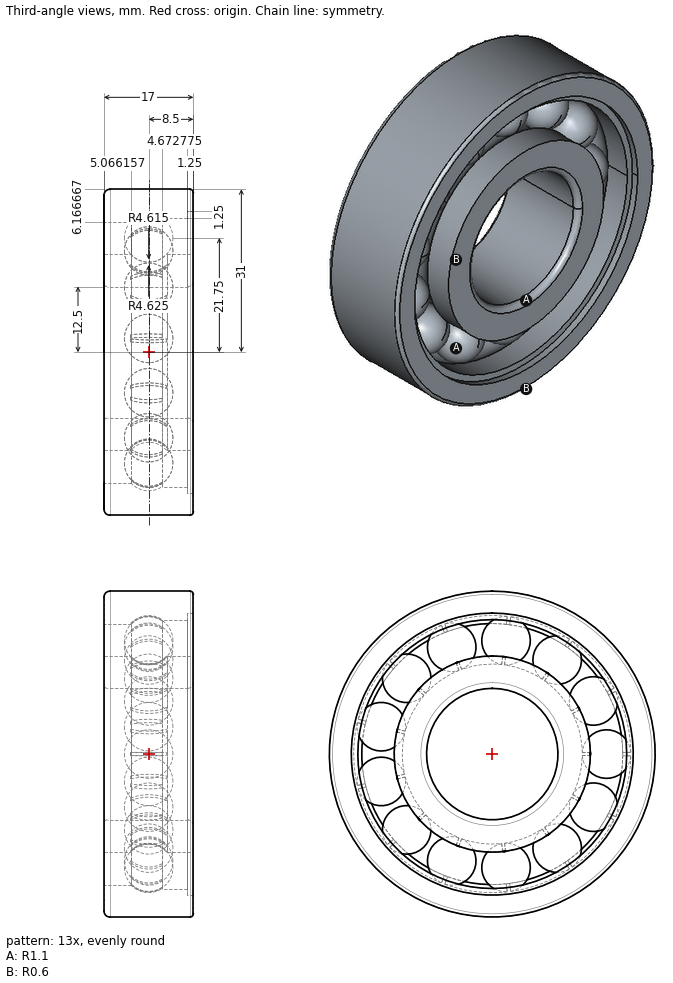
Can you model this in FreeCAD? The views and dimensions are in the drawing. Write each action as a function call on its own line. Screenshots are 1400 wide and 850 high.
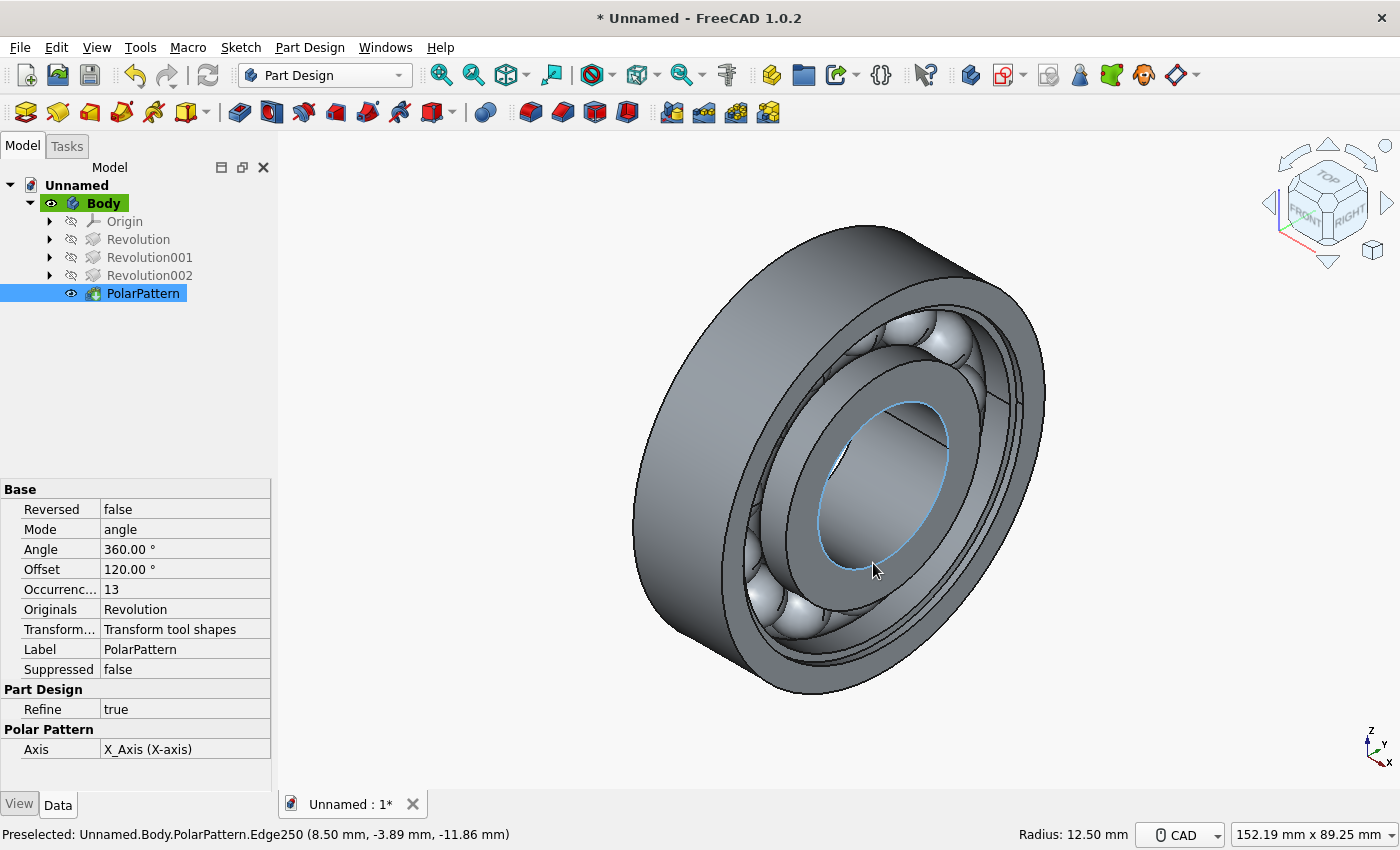
key(2)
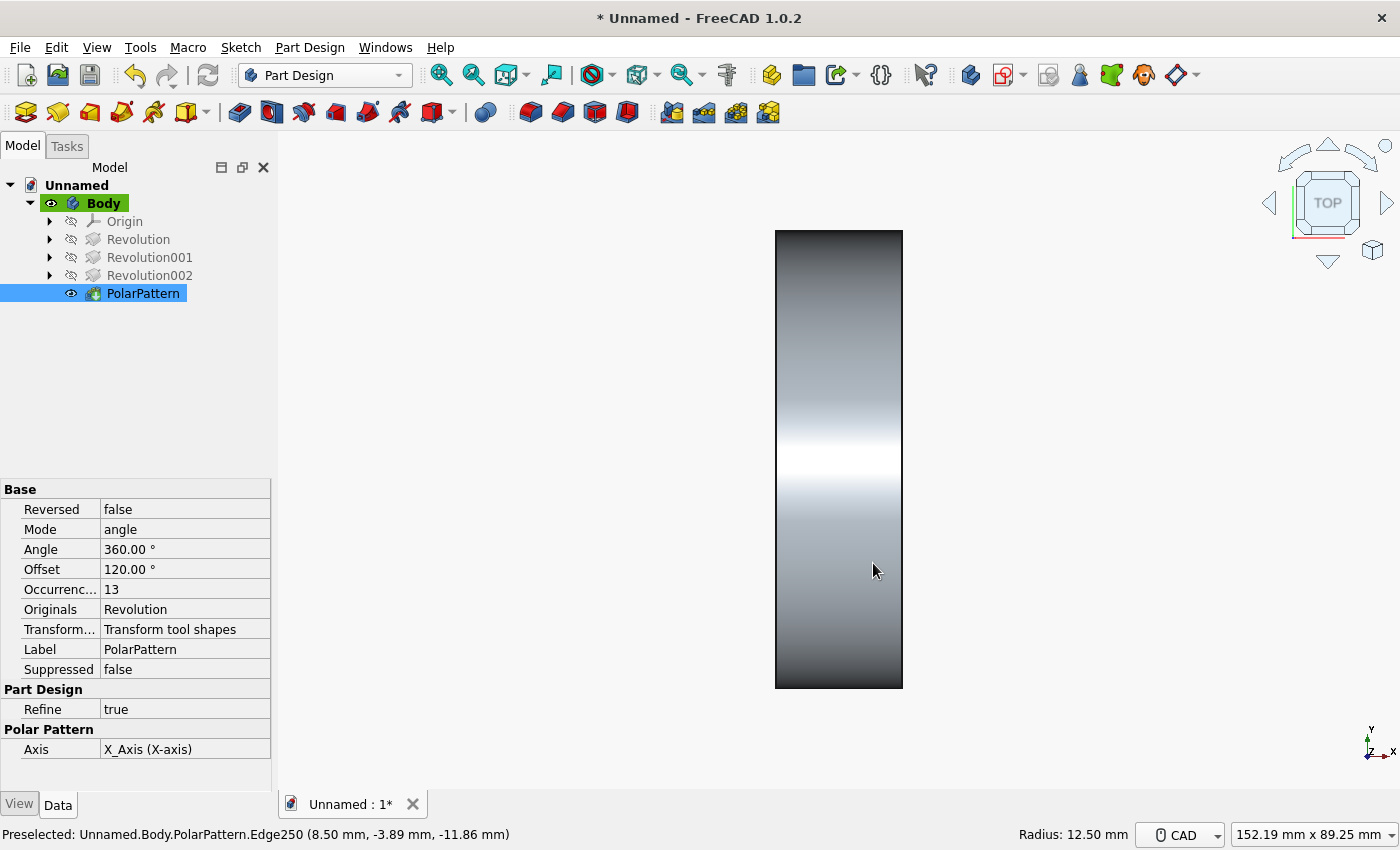
click(776, 644, ctrl)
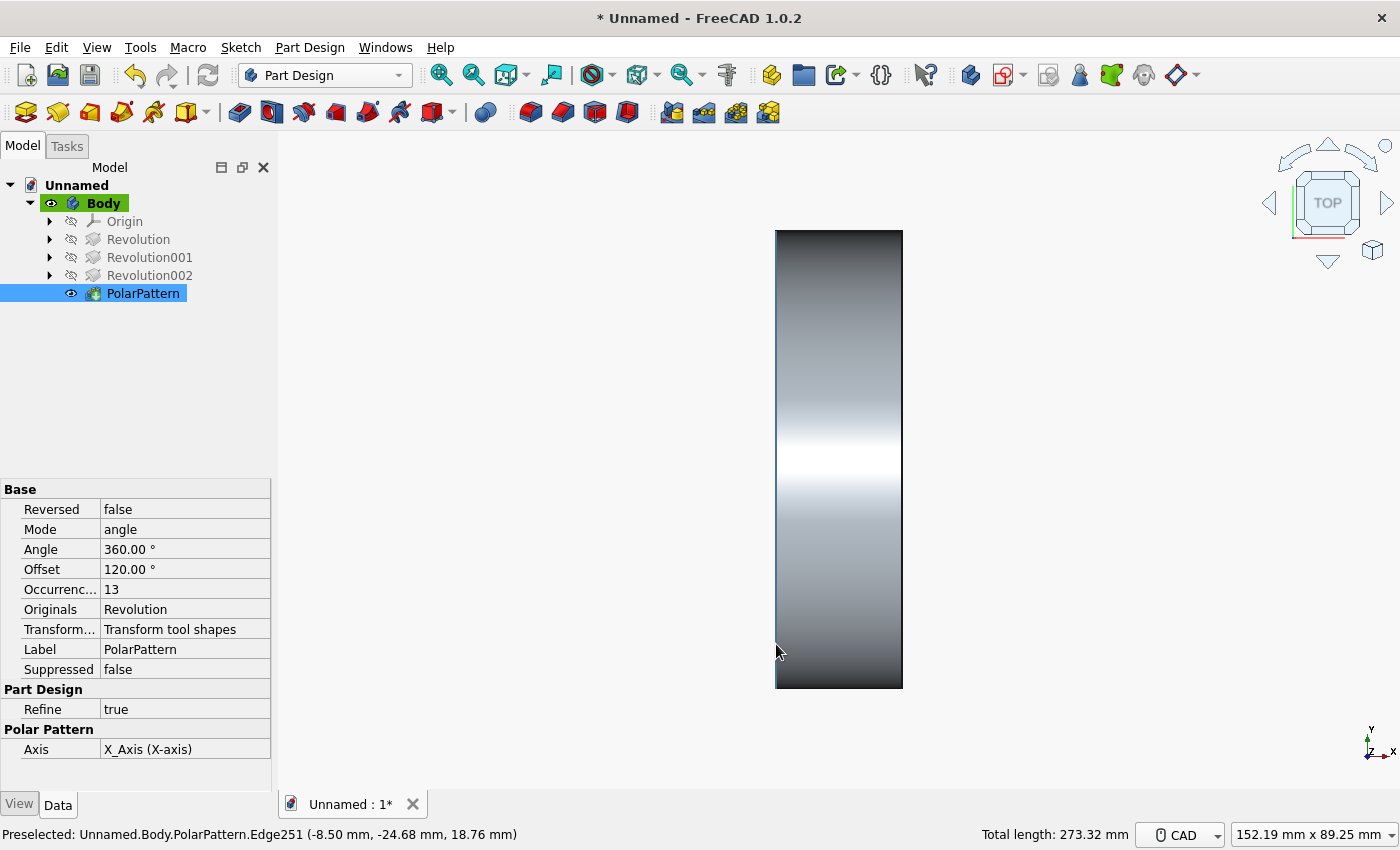
click(532, 112)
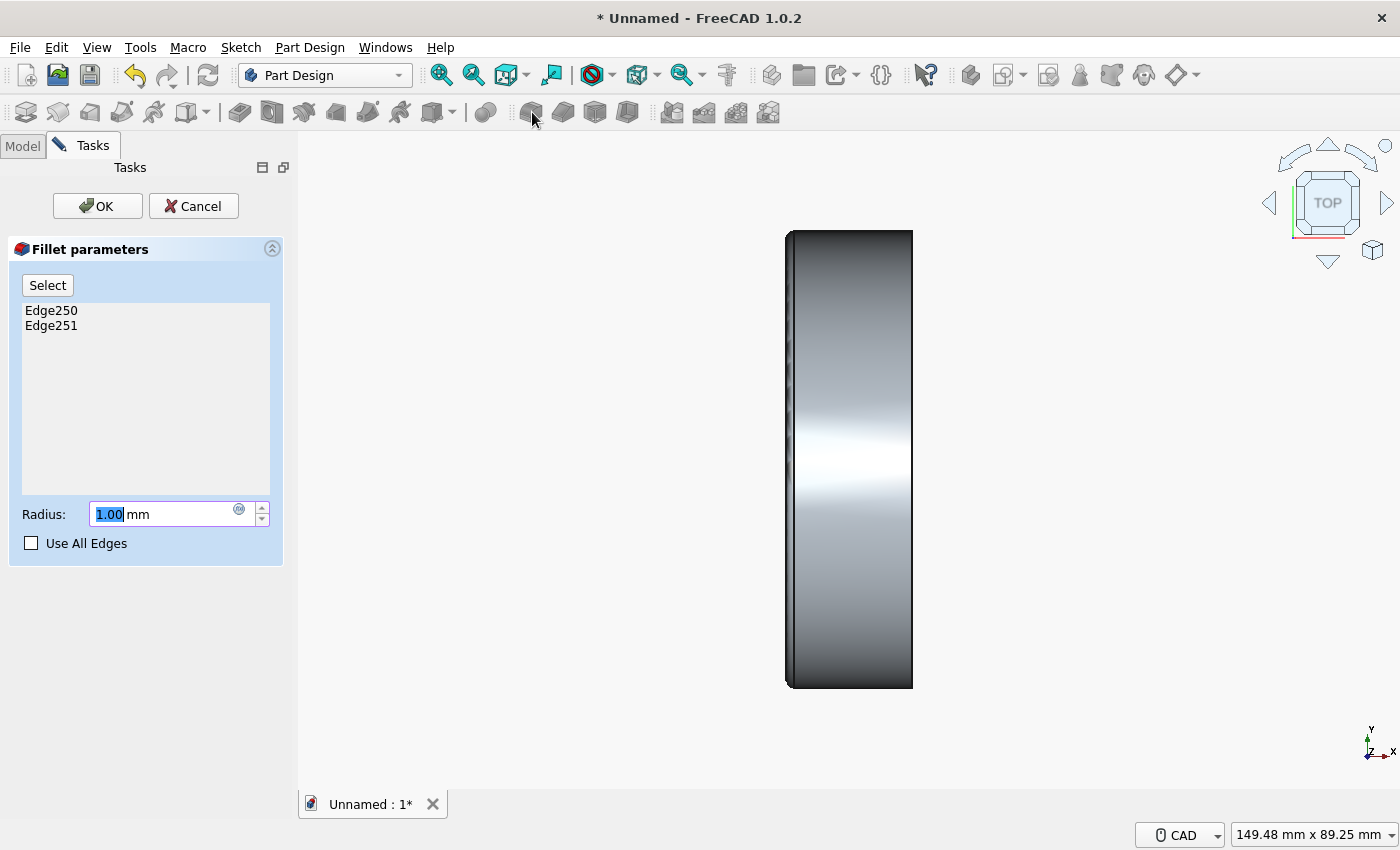
text(1.1)
key(Tab)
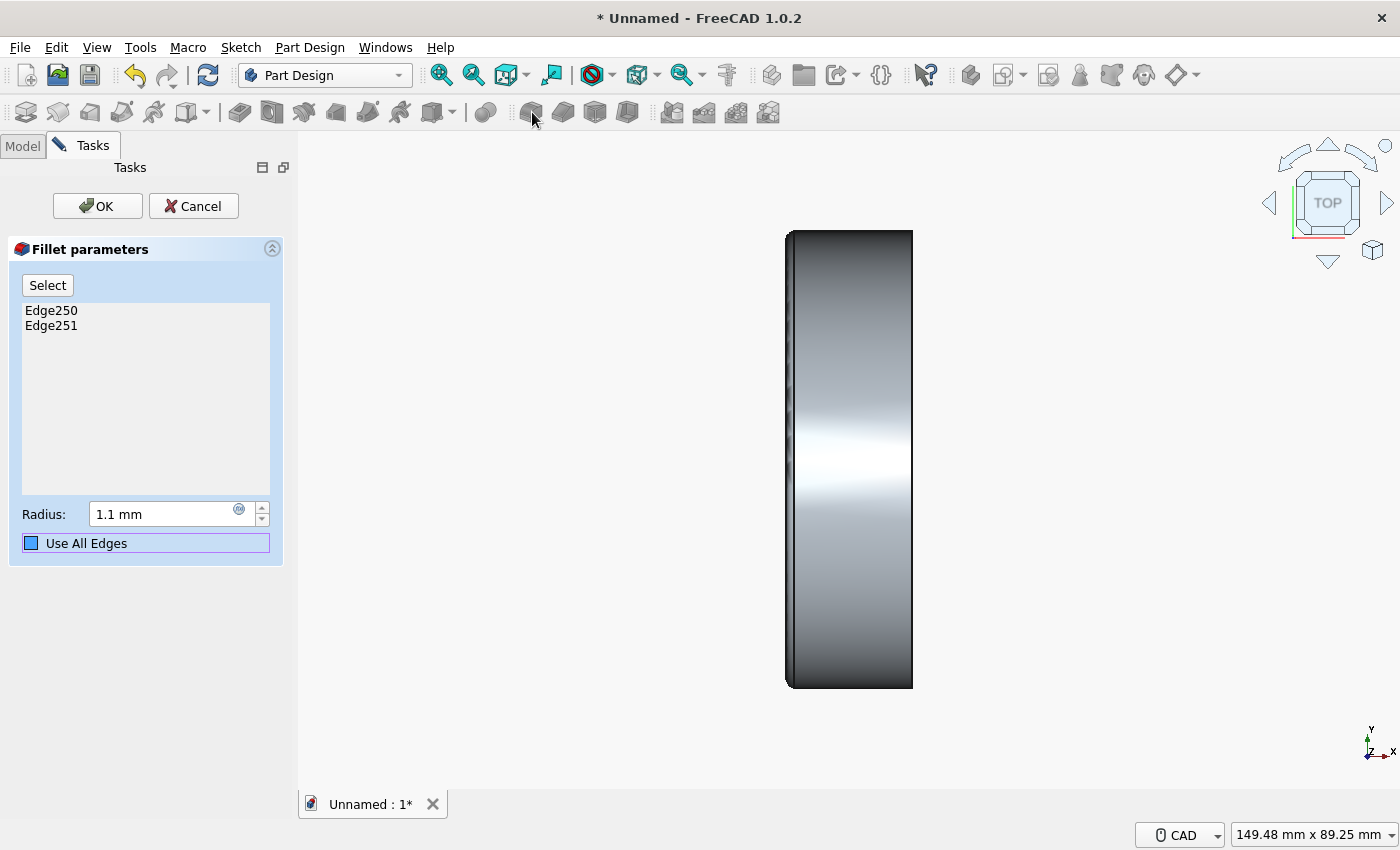
click(98, 206)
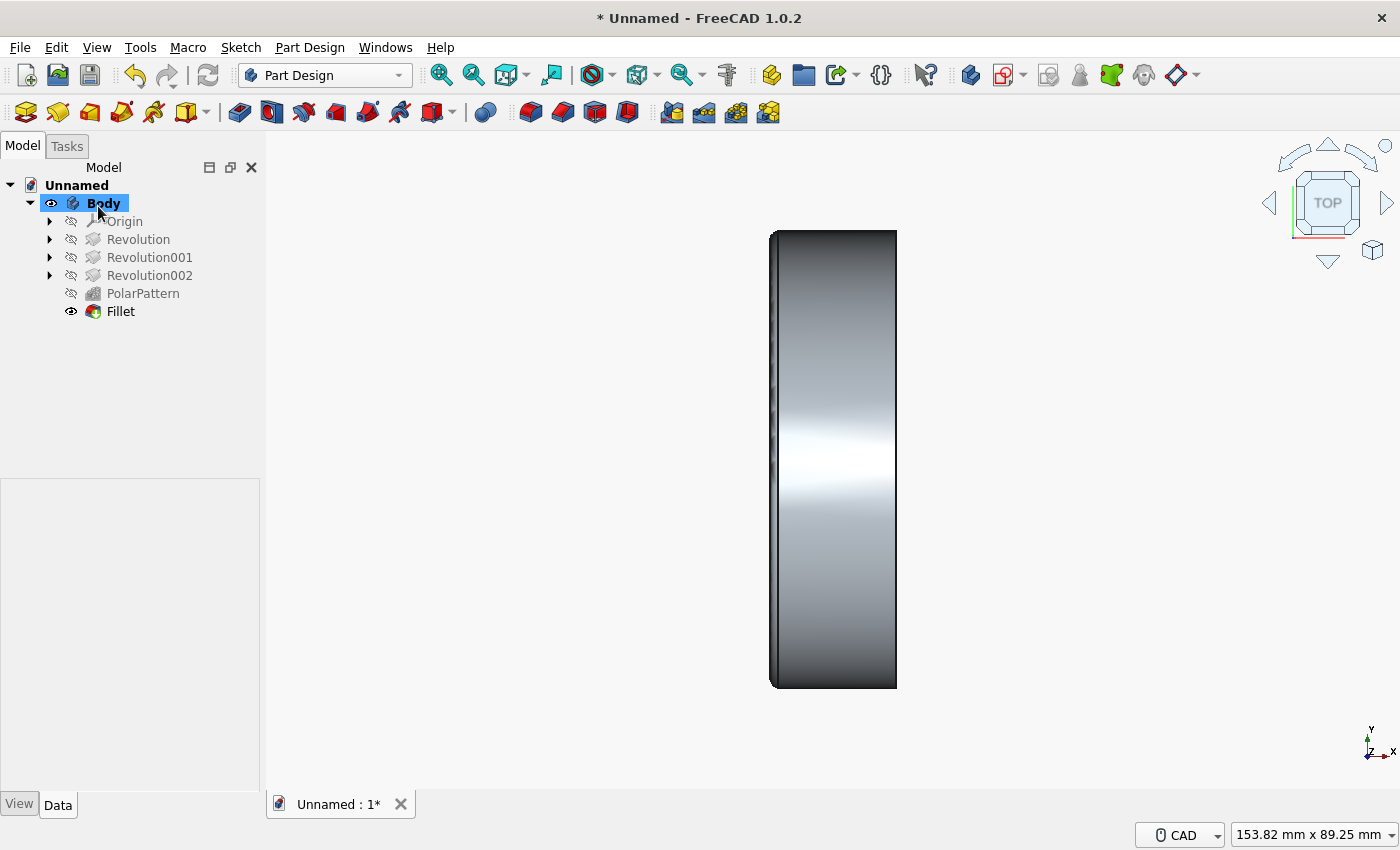
click(896, 292)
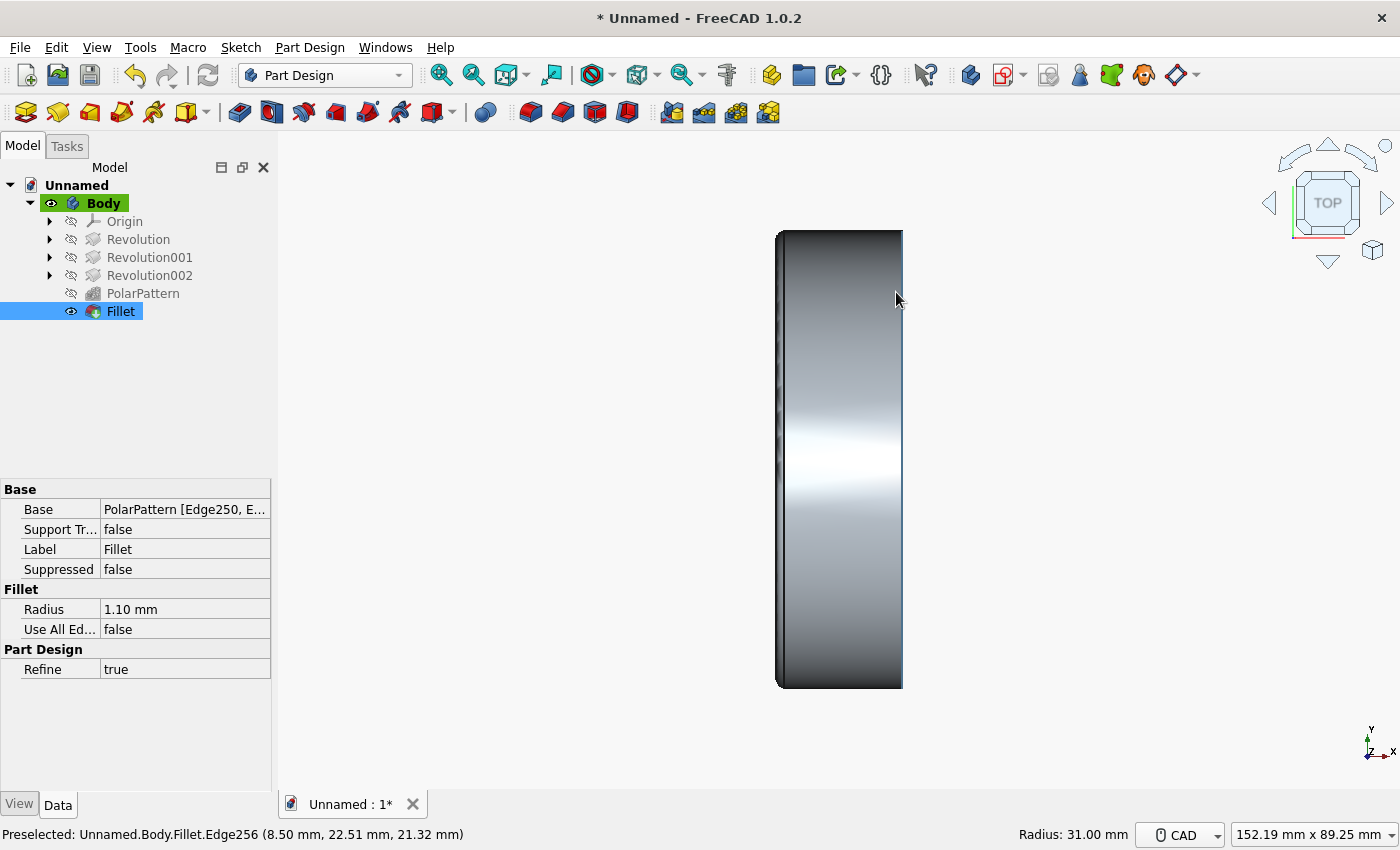
key(0)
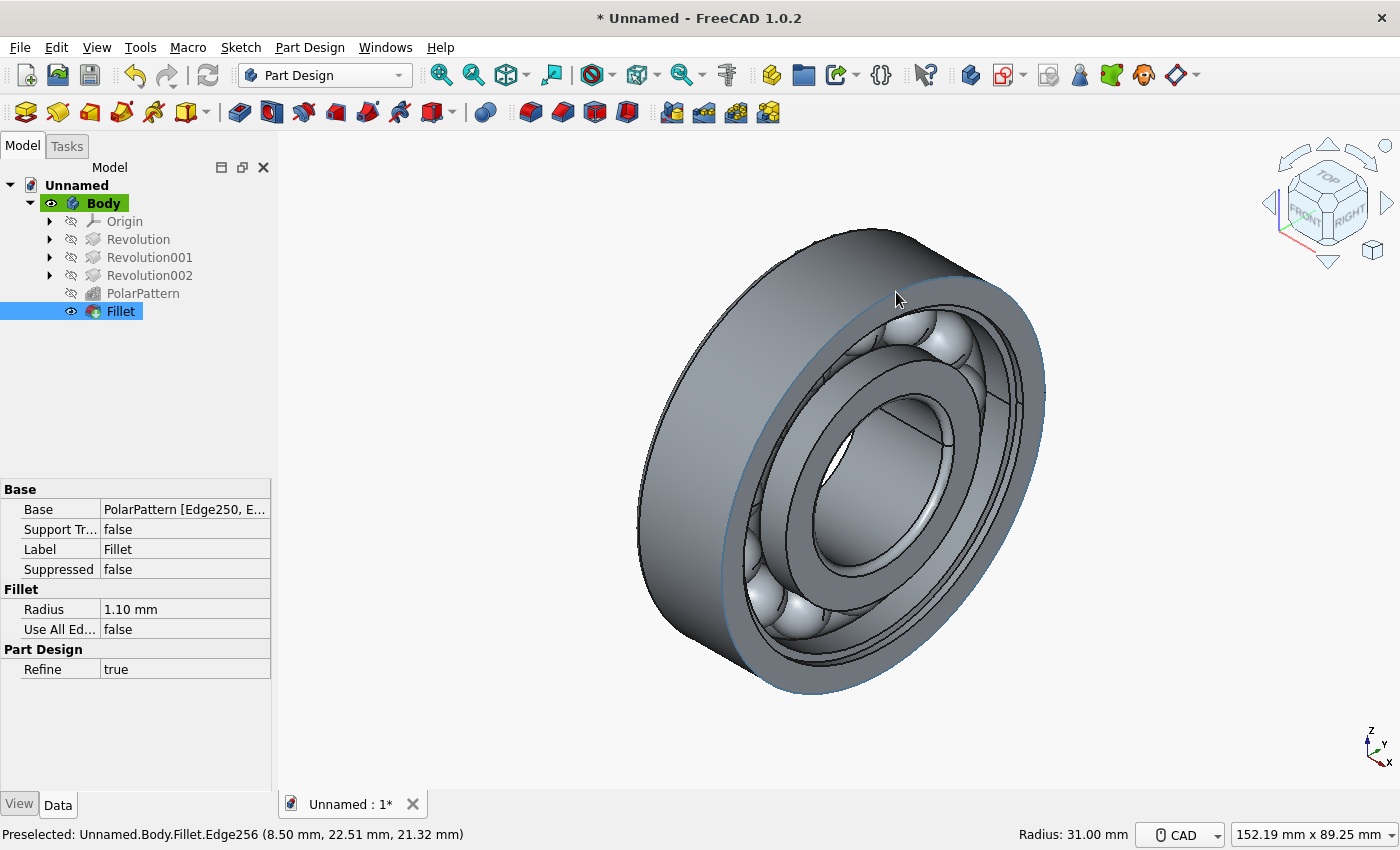
key(2)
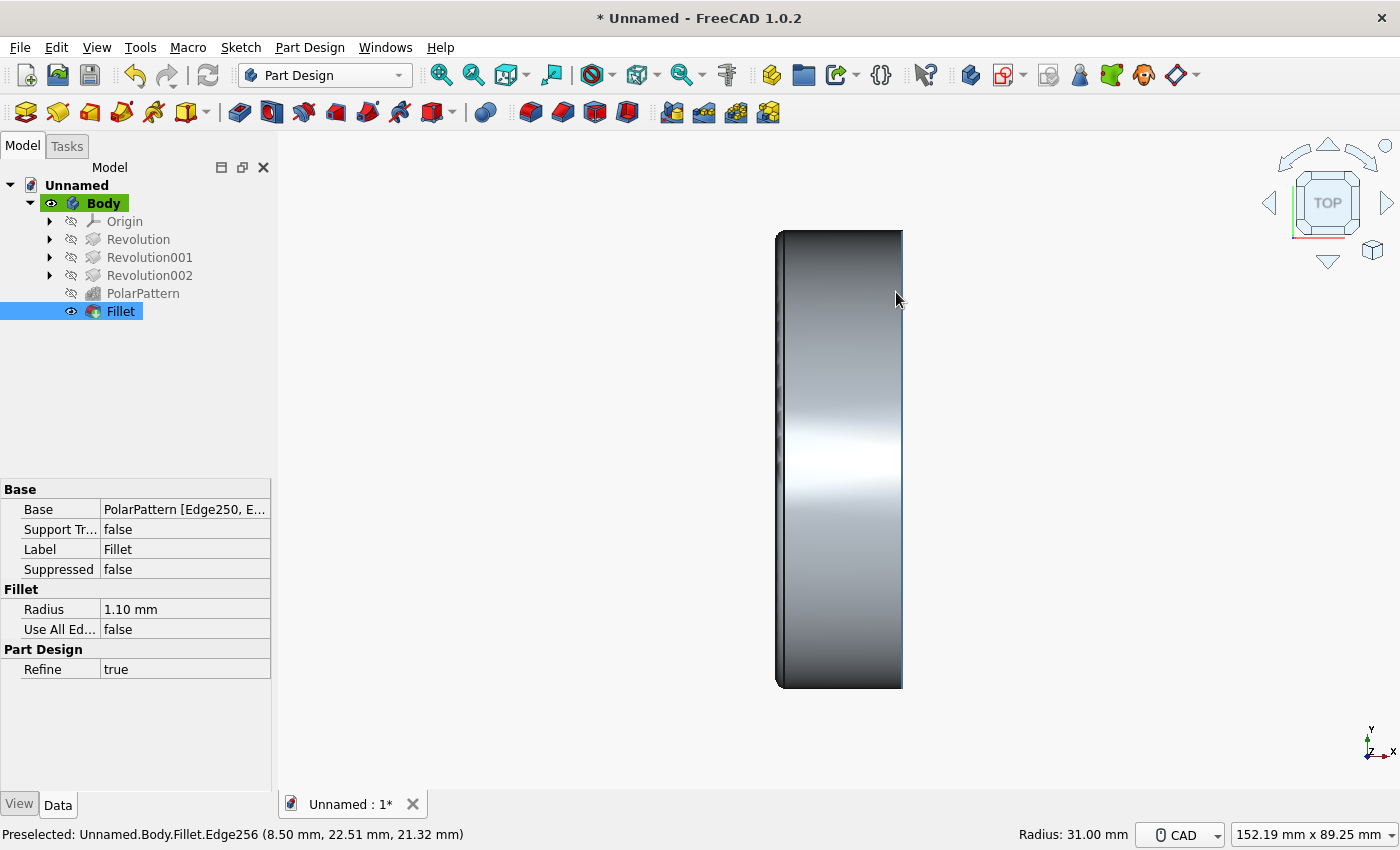
key(1)